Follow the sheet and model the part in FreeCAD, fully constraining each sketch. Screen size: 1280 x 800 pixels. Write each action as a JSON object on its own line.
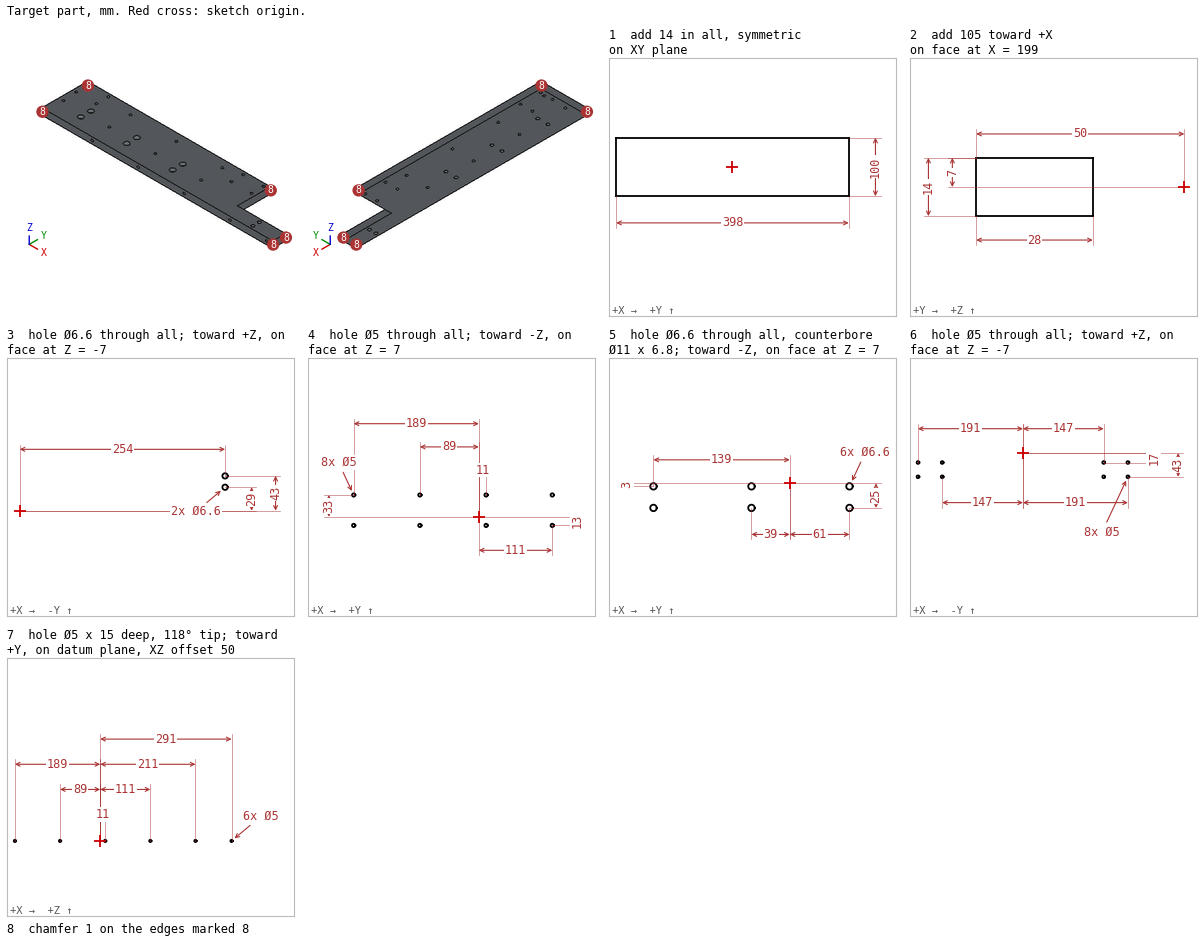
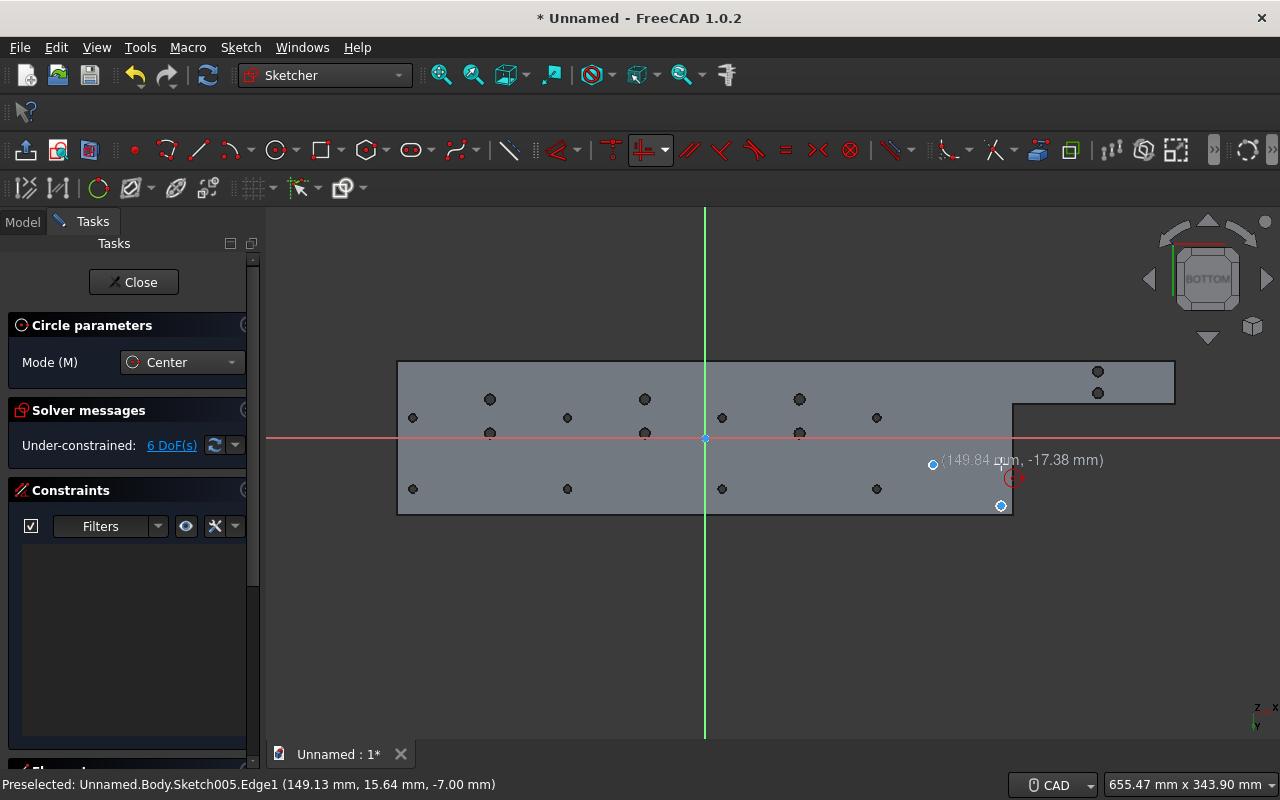
{"action": "left_click", "coordinate": [1001, 464]}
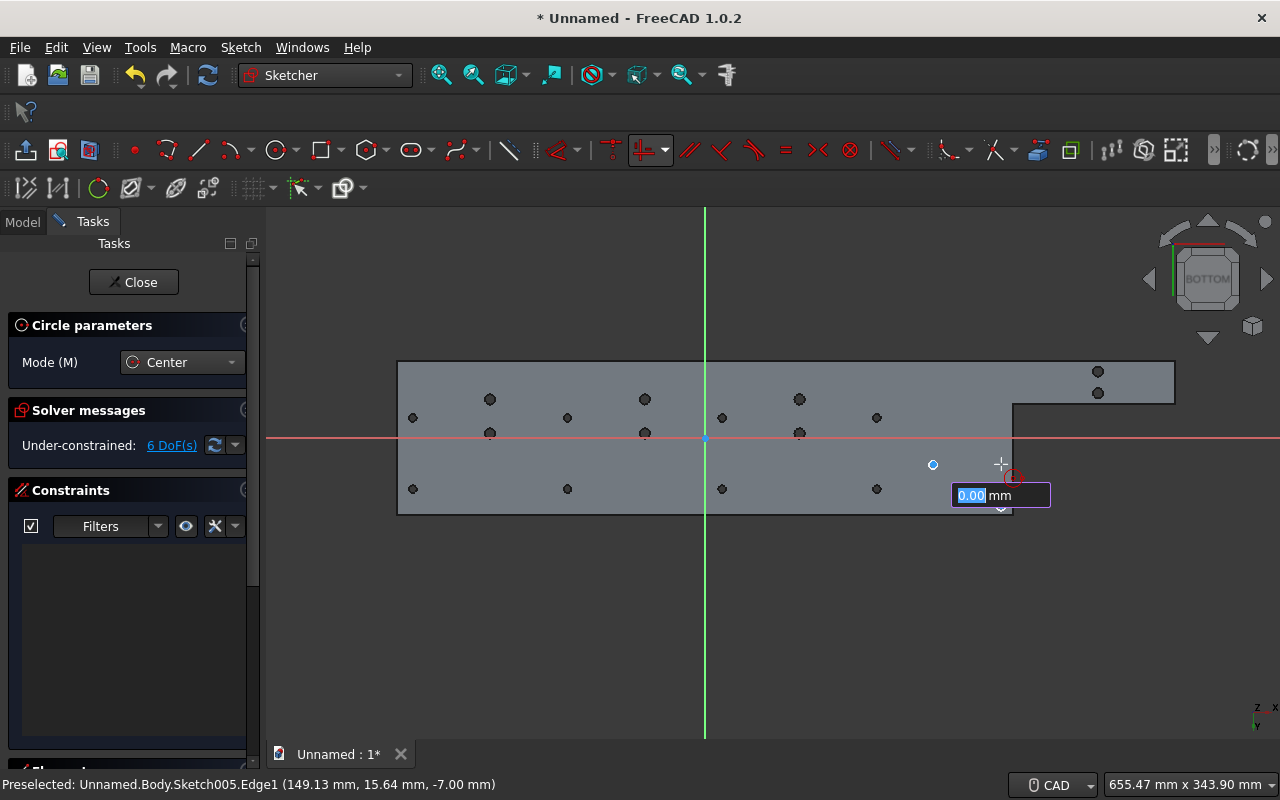
{"action": "scroll", "coordinate": [1003, 462], "scroll_direction": "up", "scroll_amount": 8}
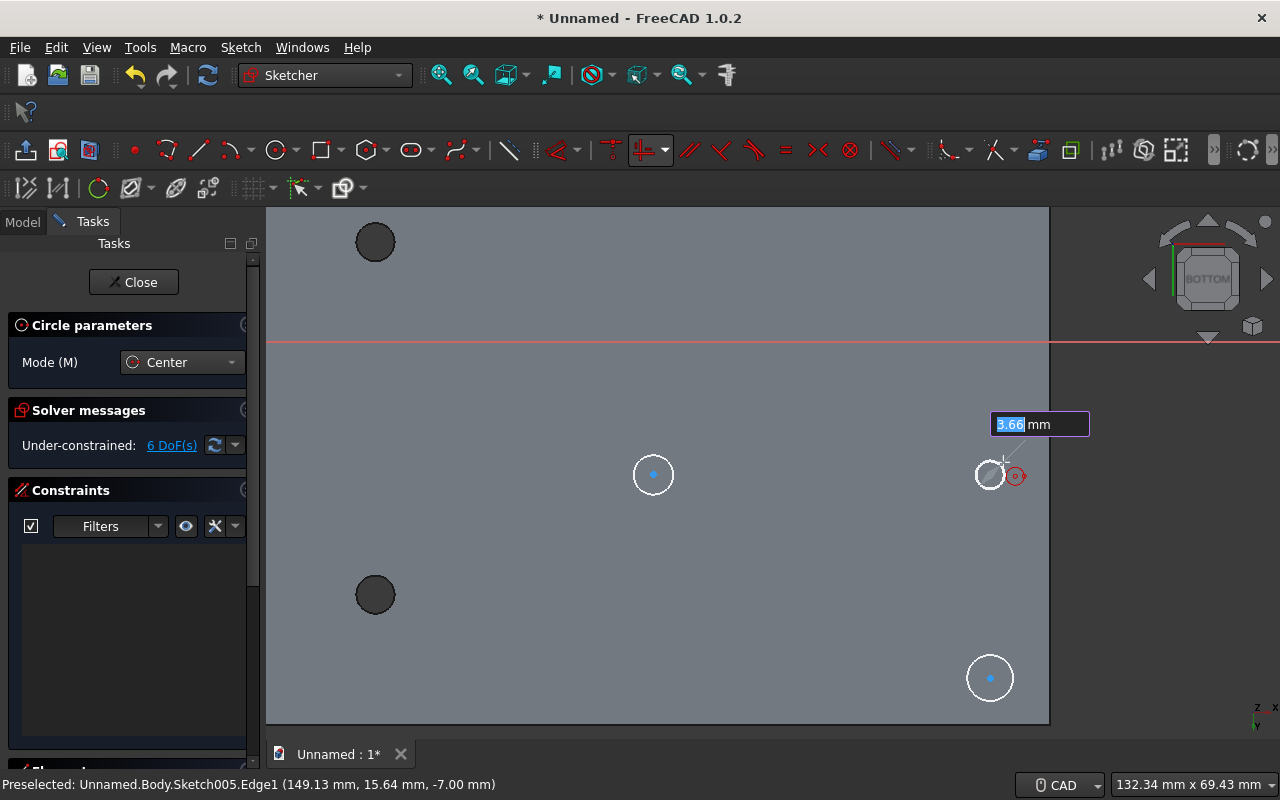
{"action": "left_click", "coordinate": [1002, 458]}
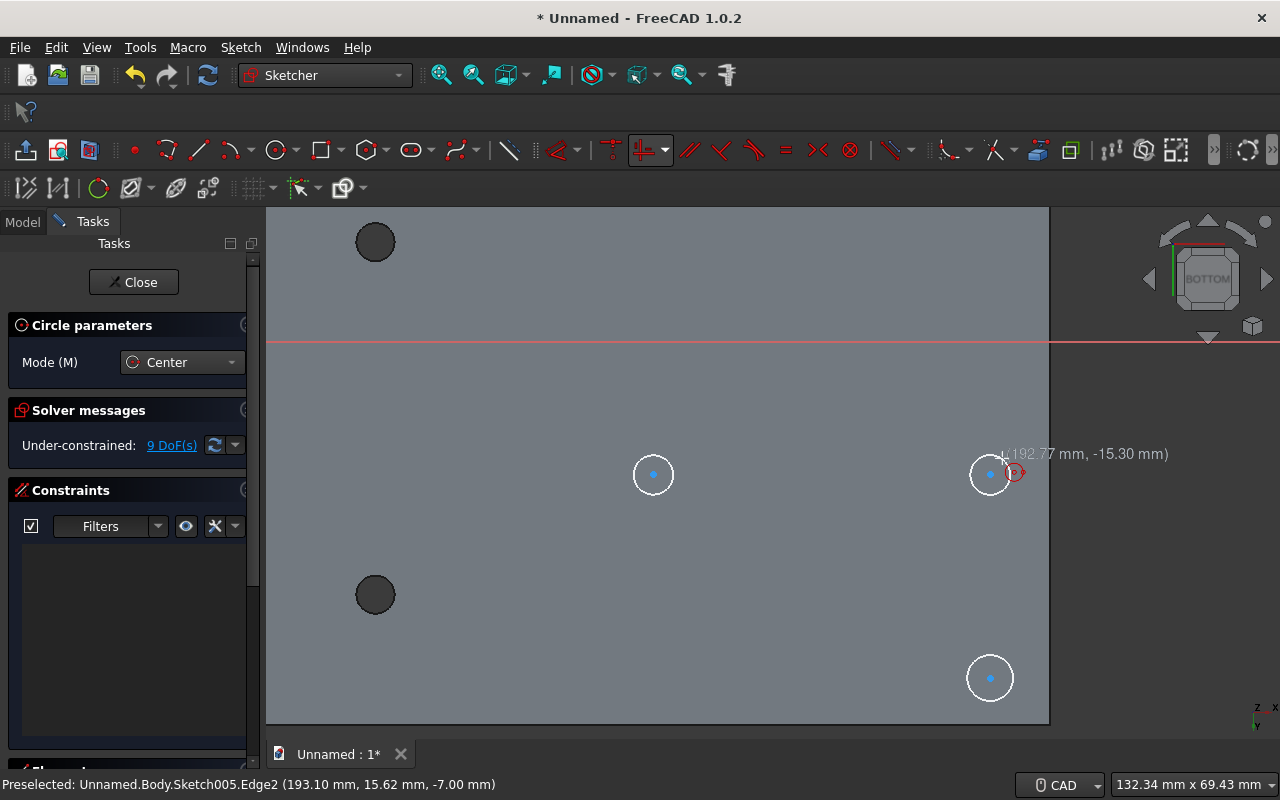
{"action": "scroll", "coordinate": [1003, 462], "scroll_direction": "down", "scroll_amount": 8}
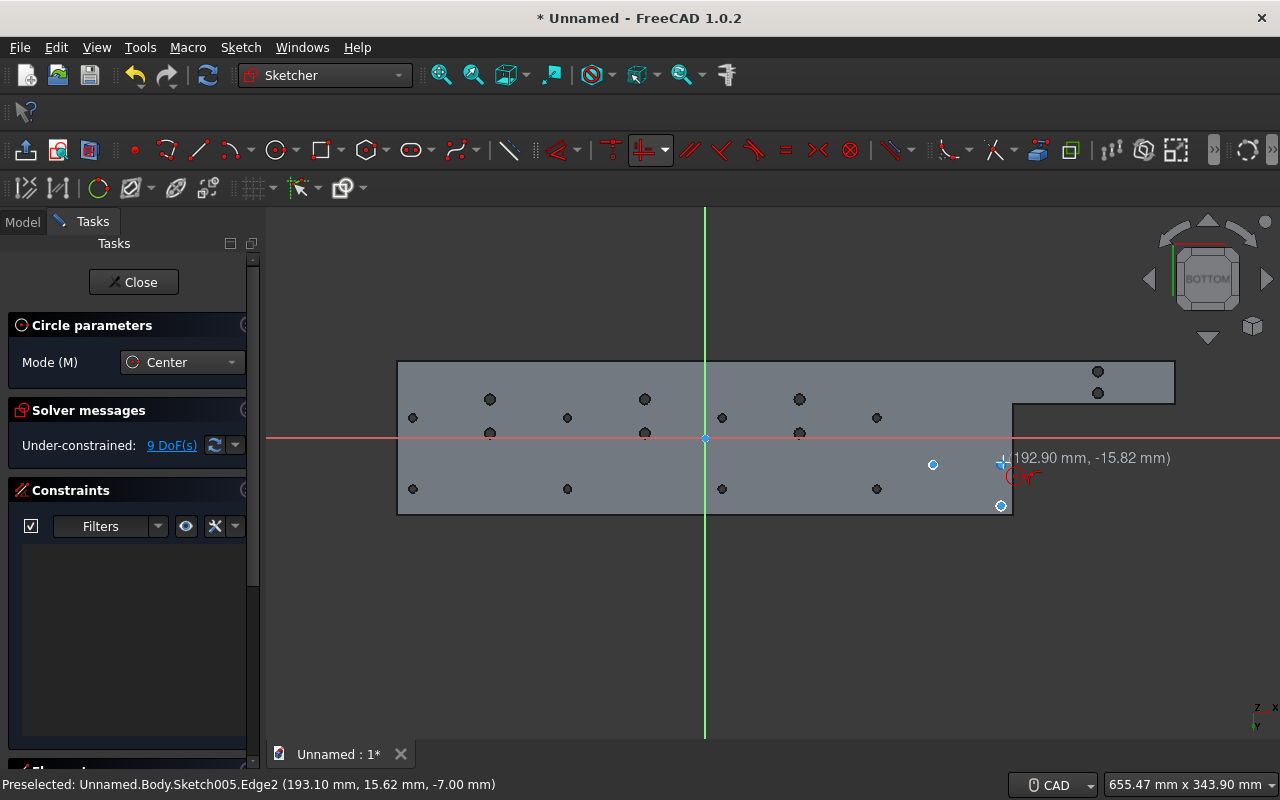
{"action": "left_click", "coordinate": [933, 505]}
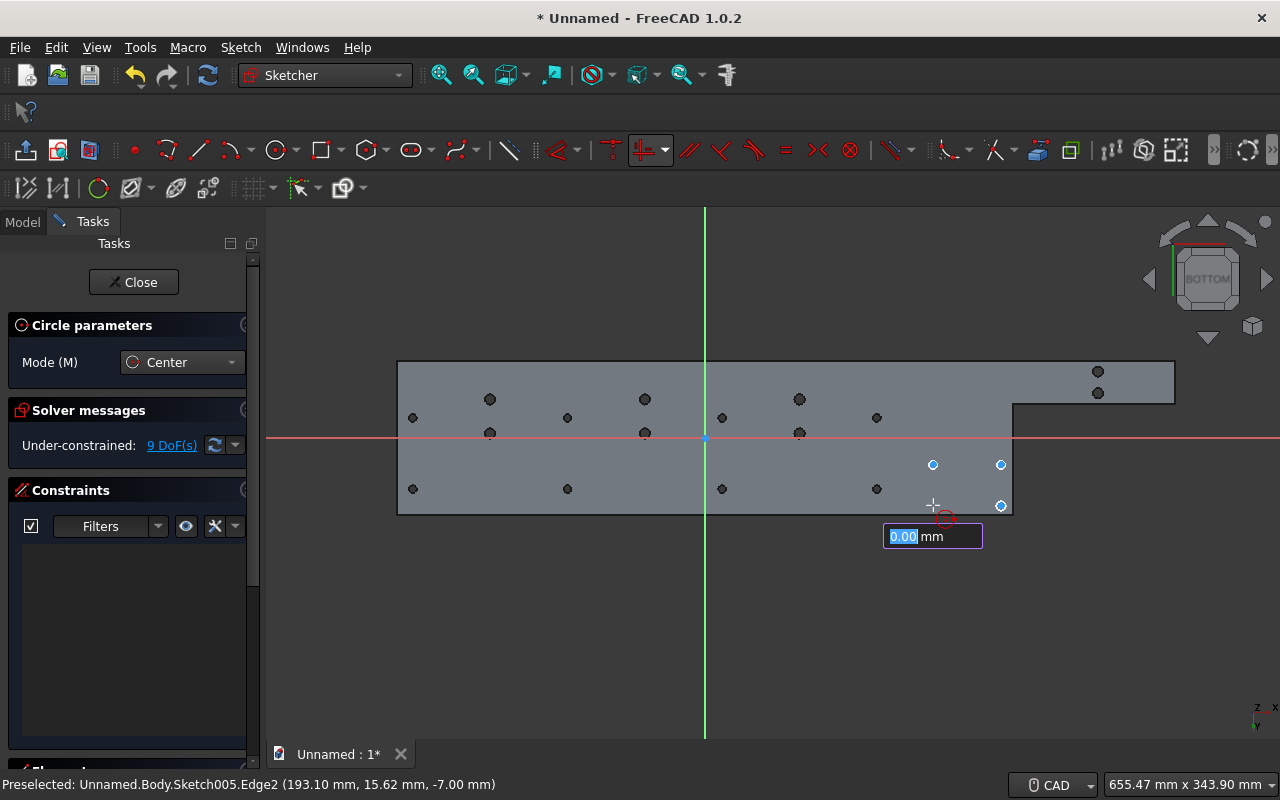
{"action": "scroll", "coordinate": [935, 502], "scroll_direction": "up", "scroll_amount": 8}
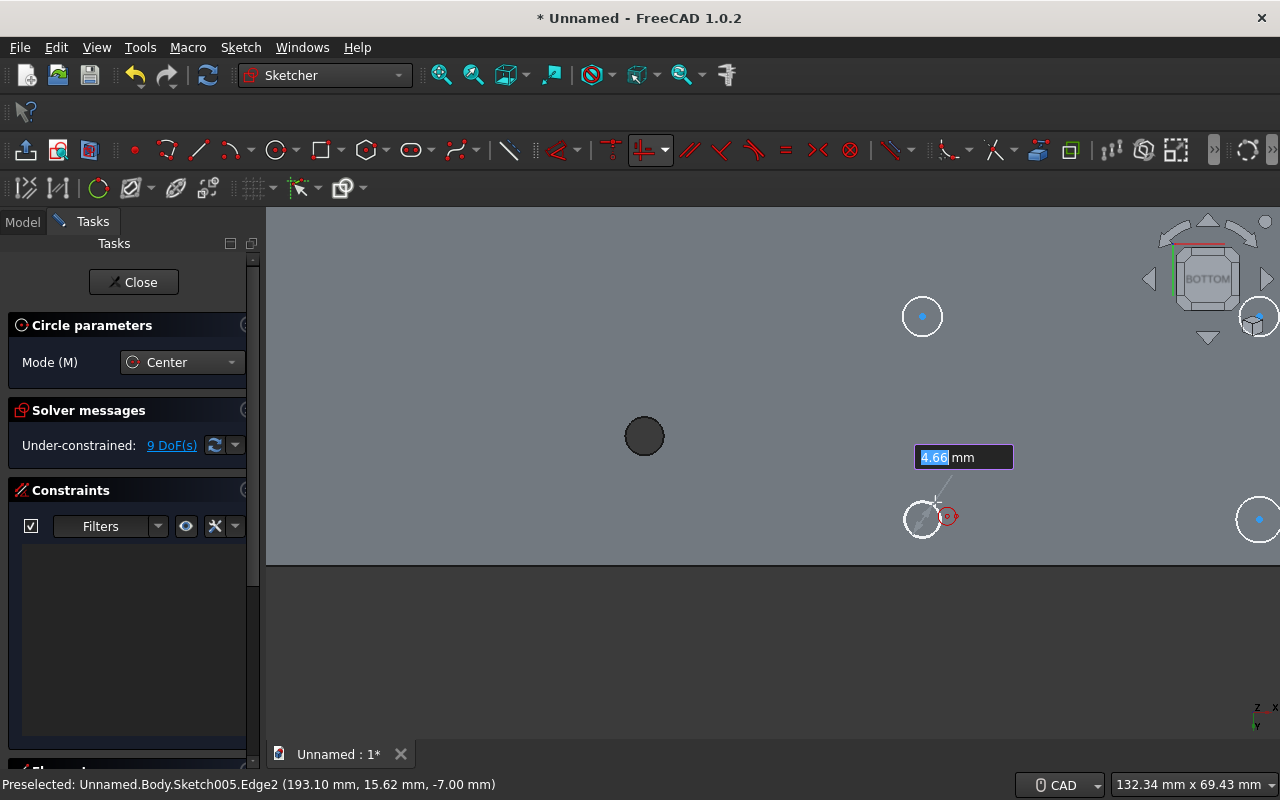
{"action": "left_click", "coordinate": [934, 499]}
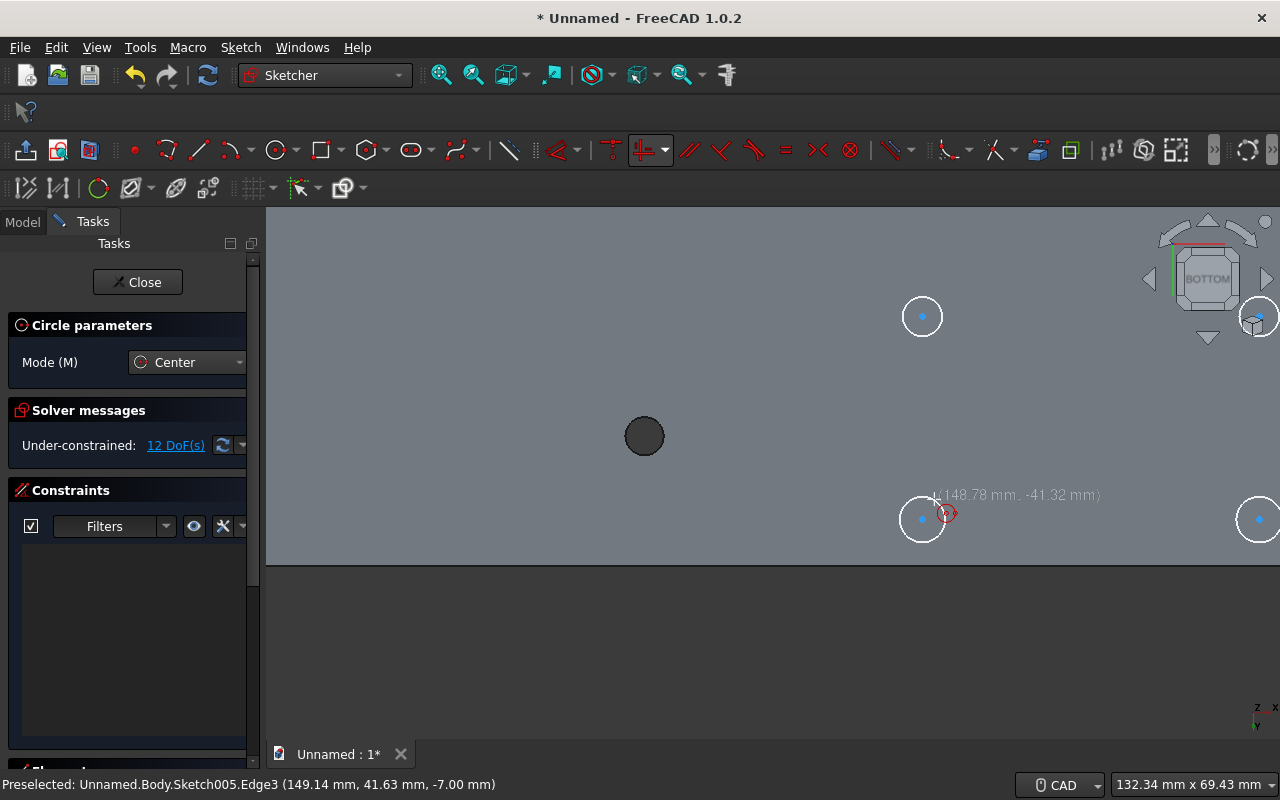
{"action": "scroll", "coordinate": [935, 502], "scroll_direction": "down", "scroll_amount": 8}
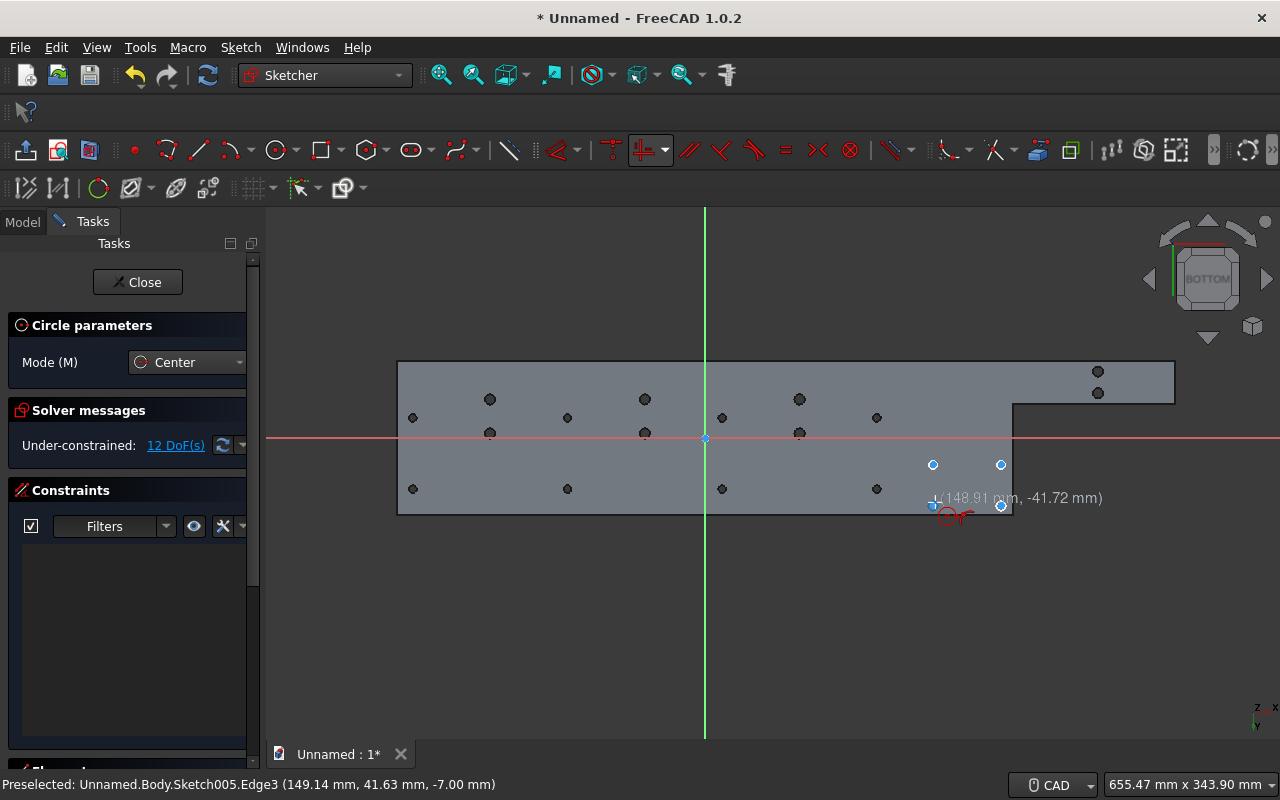
{"action": "scroll", "coordinate": [478, 505], "scroll_direction": "up", "scroll_amount": 9}